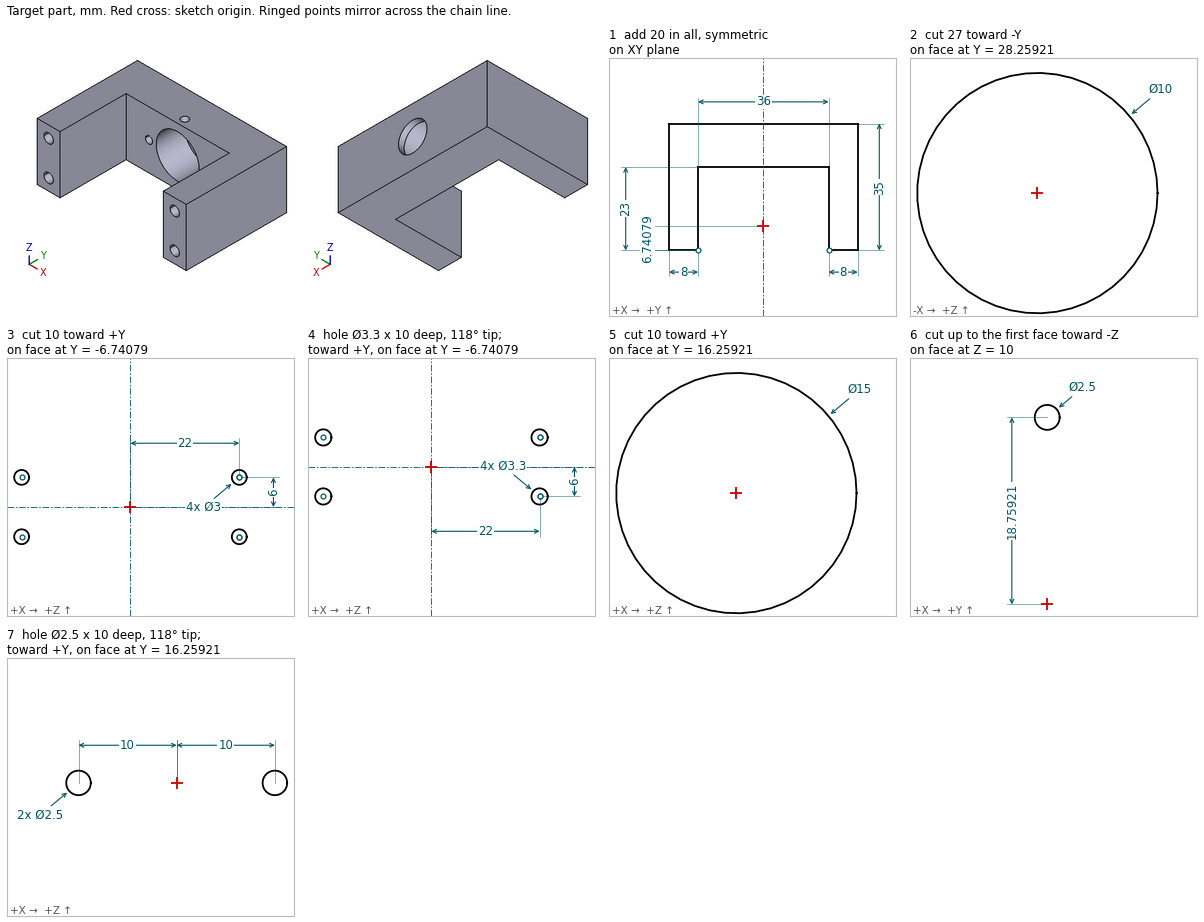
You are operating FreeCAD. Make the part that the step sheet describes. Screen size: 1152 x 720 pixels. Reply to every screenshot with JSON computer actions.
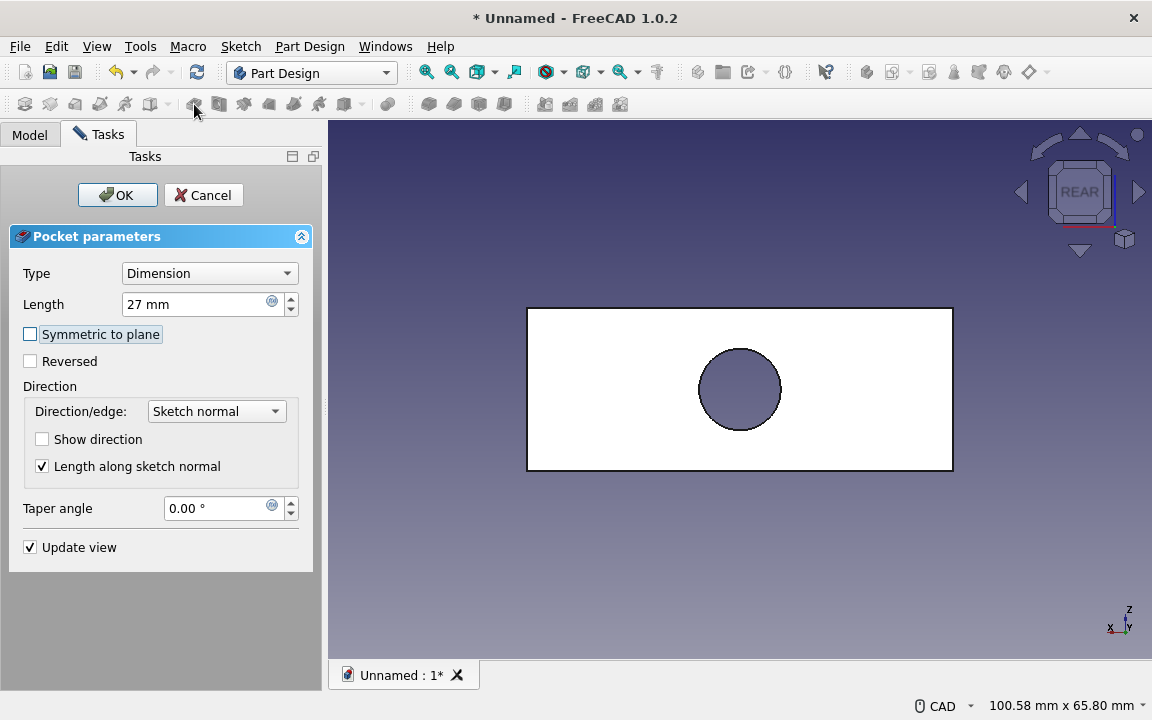
{"action": "left_click", "coordinate": [118, 195]}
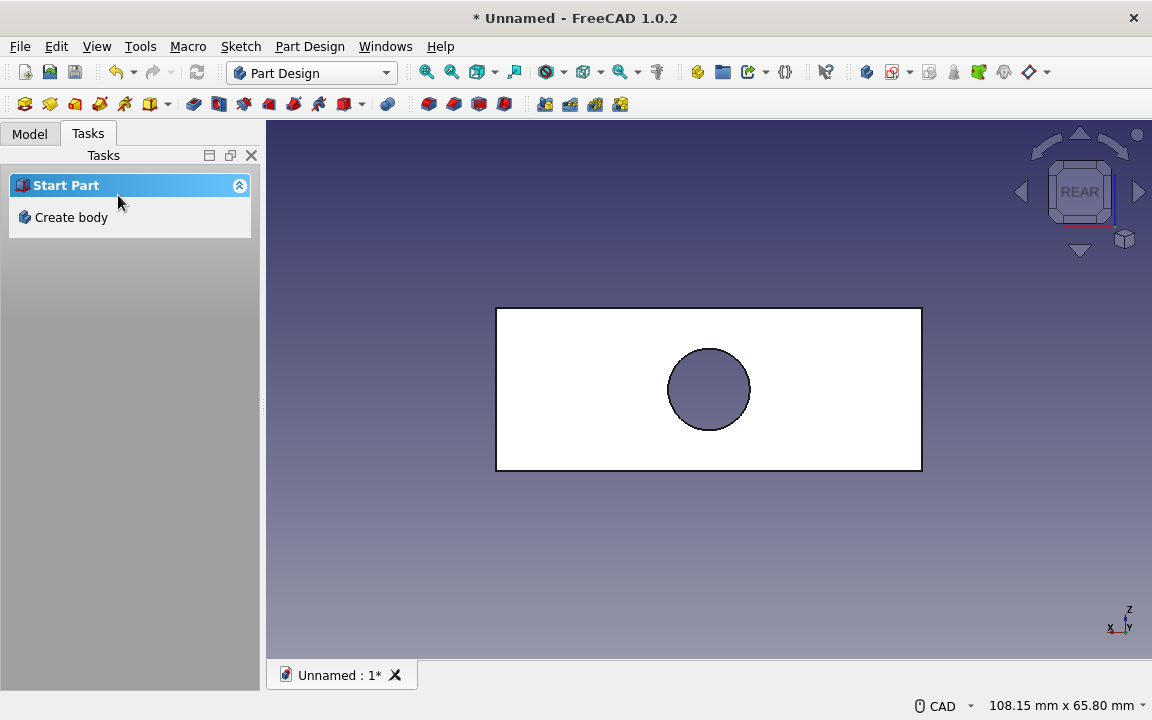
{"action": "key", "text": "0"}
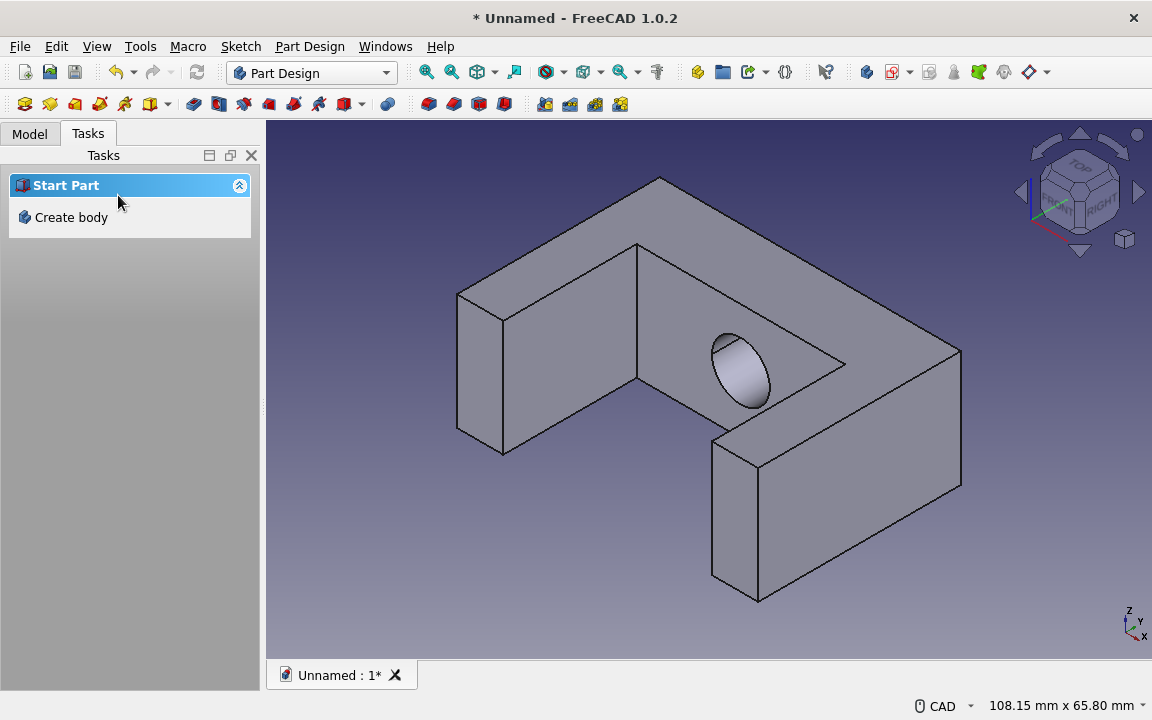
{"action": "left_click", "coordinate": [735, 482]}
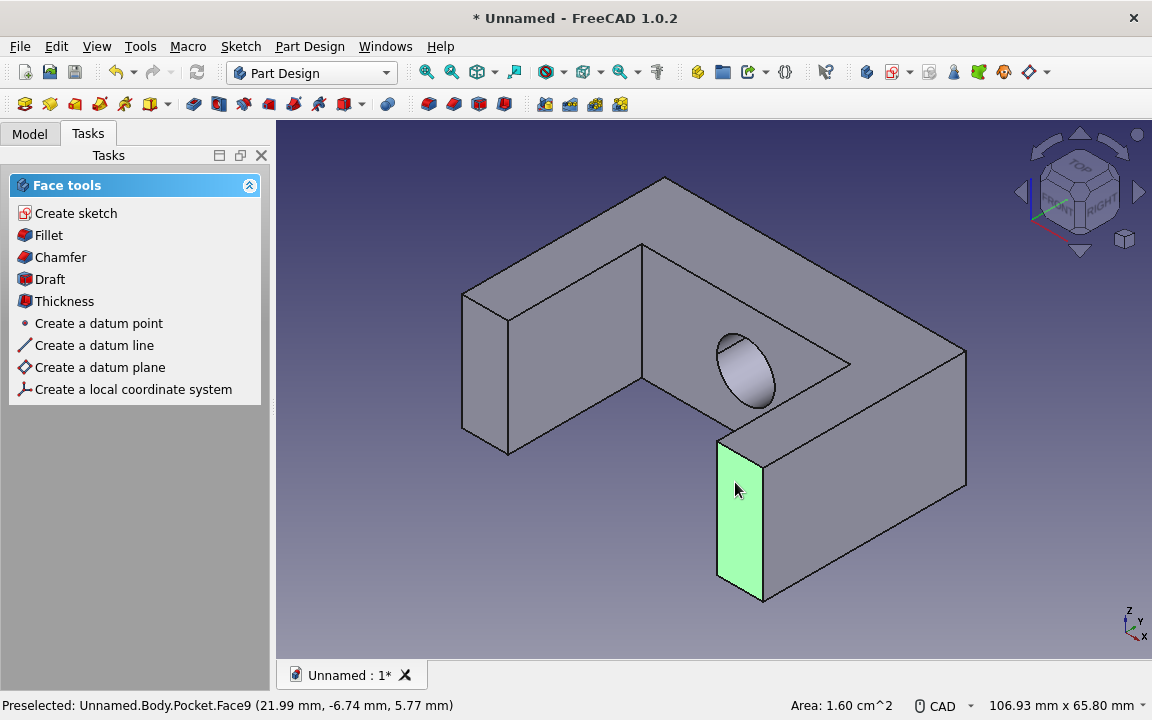
{"action": "left_click", "coordinate": [892, 72]}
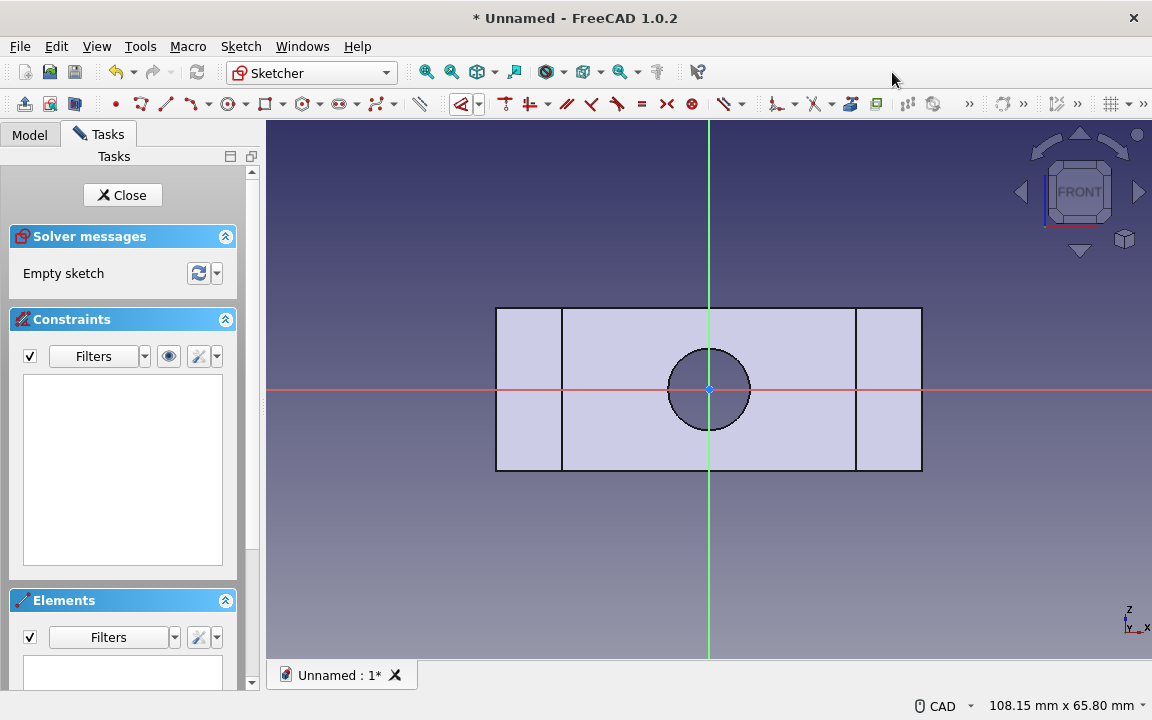
{"action": "key", "text": "g c"}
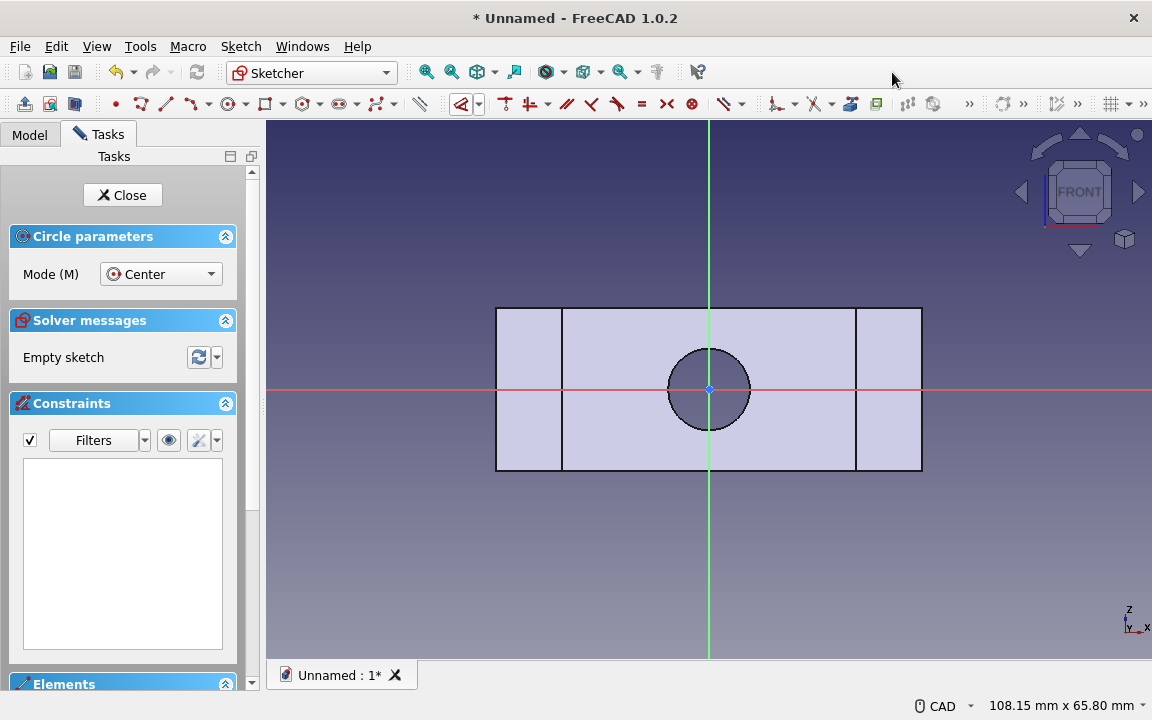
{"action": "scroll", "coordinate": [889, 340], "scroll_direction": "up", "scroll_amount": 4}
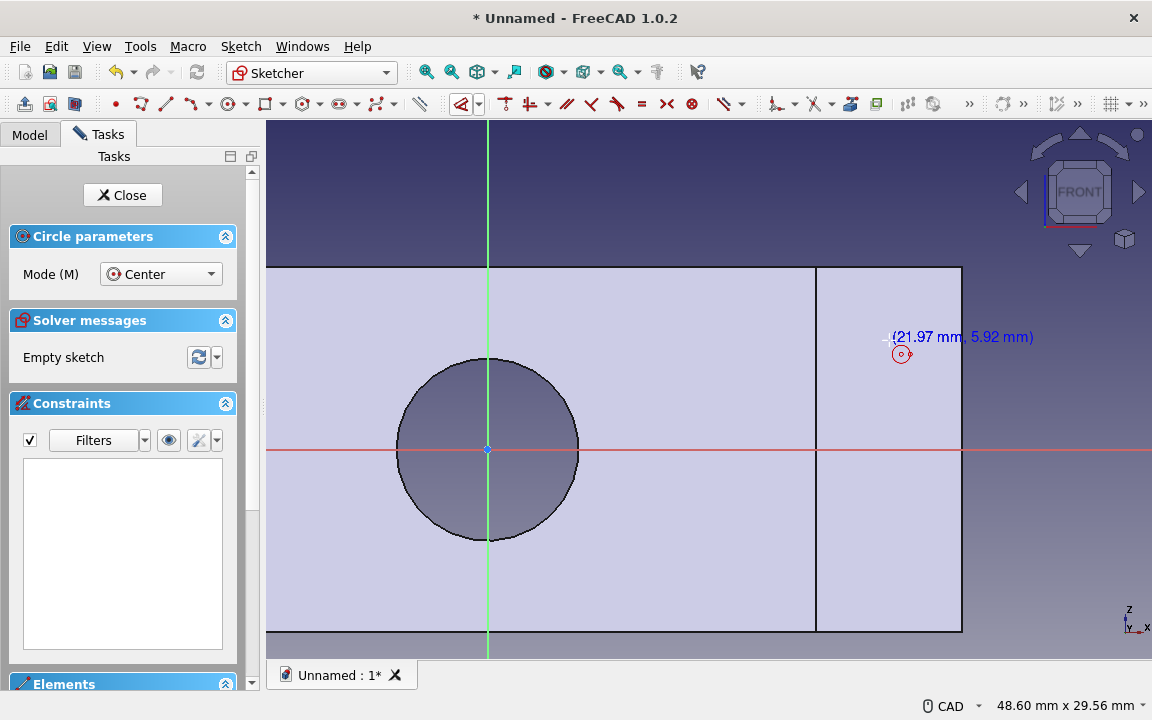
{"action": "left_click", "coordinate": [889, 340]}
{"action": "left_click", "coordinate": [908, 321]}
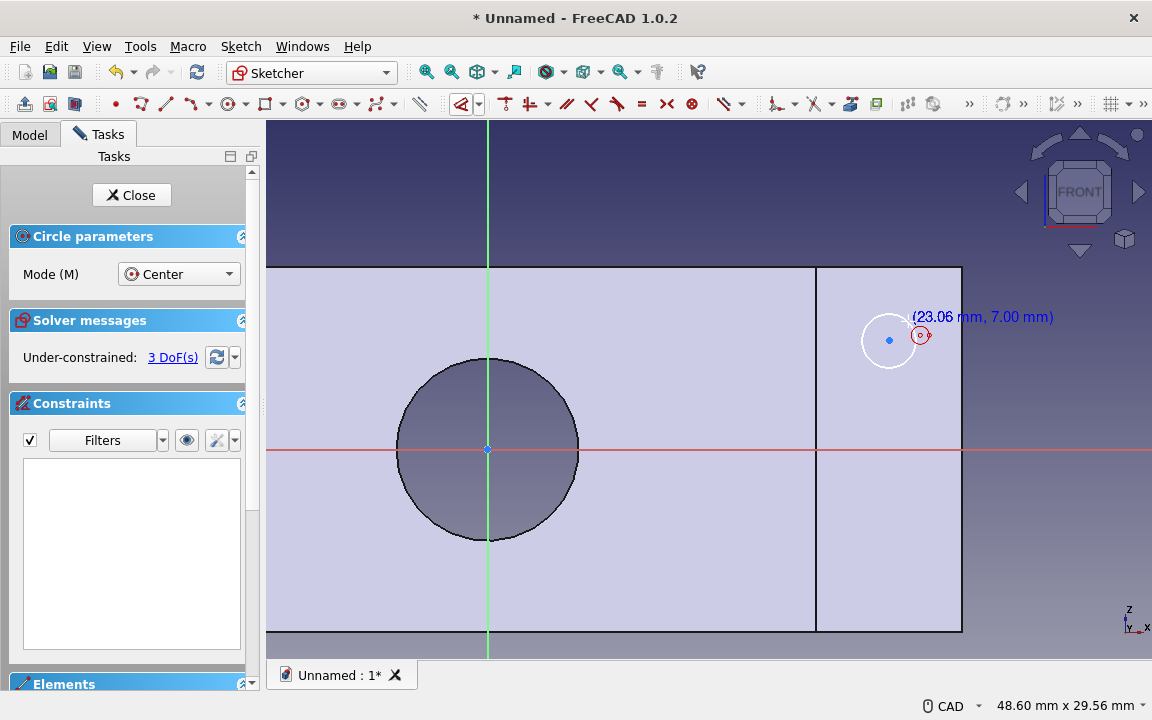
{"action": "left_click", "coordinate": [889, 559]}
{"action": "left_click", "coordinate": [908, 540]}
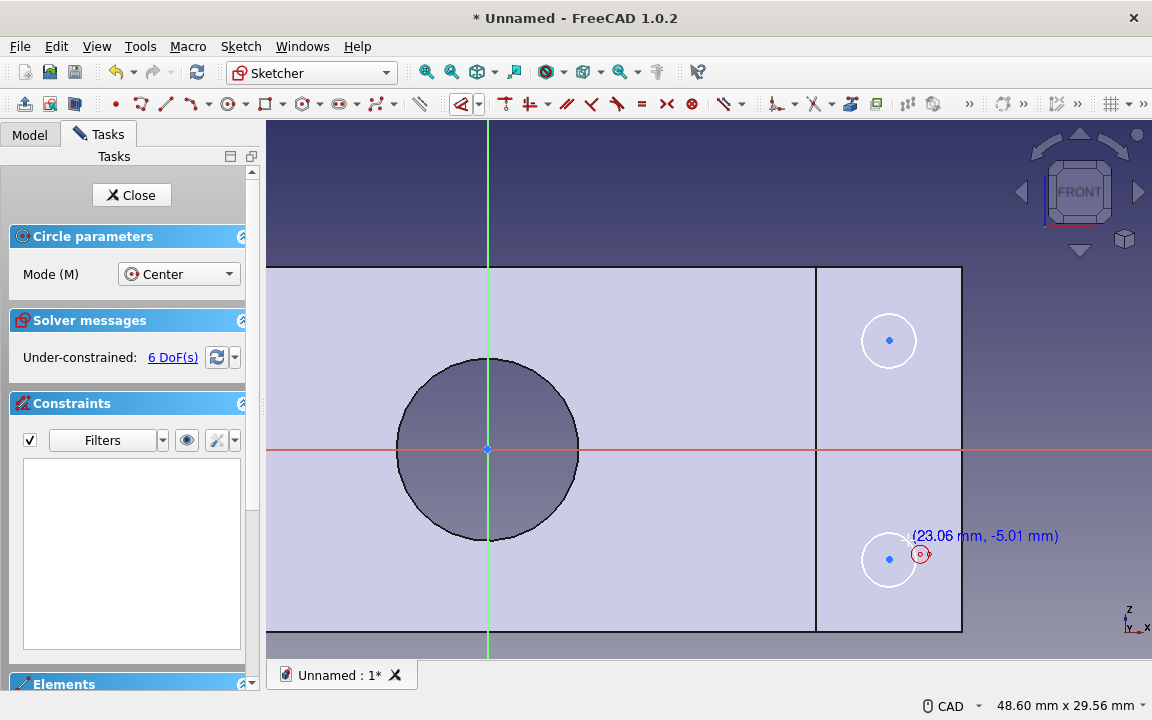
{"action": "scroll", "coordinate": [827, 316], "scroll_direction": "down", "scroll_amount": 3}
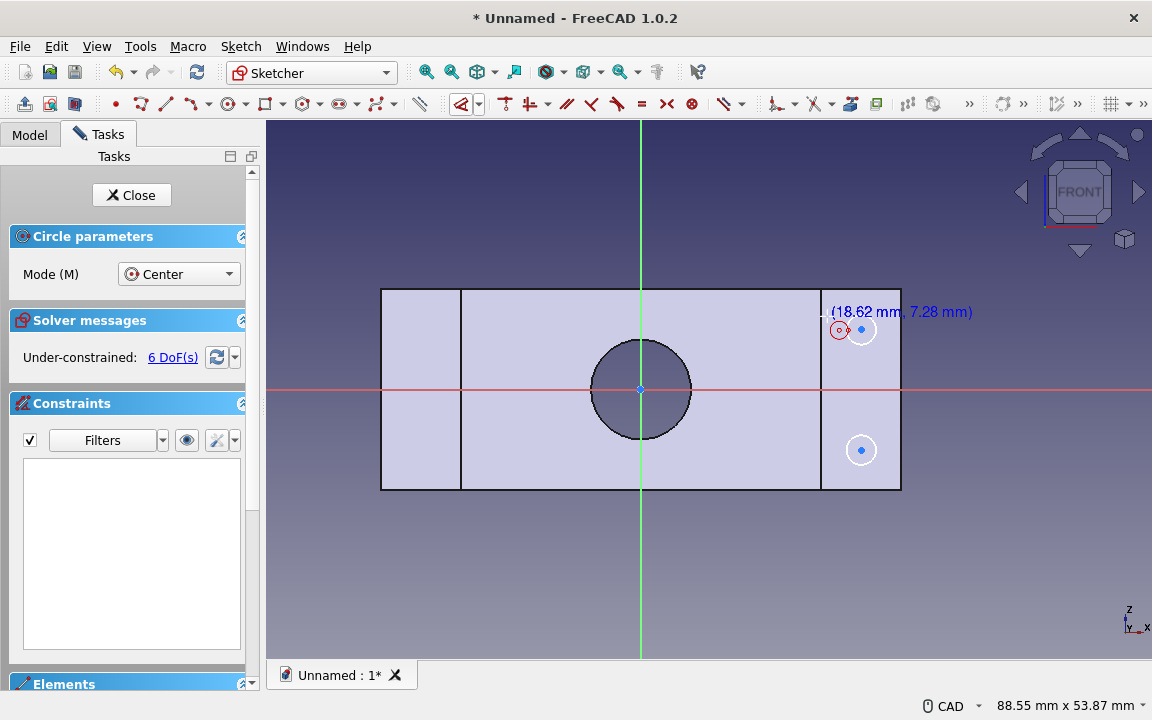
{"action": "scroll", "coordinate": [421, 450], "scroll_direction": "up", "scroll_amount": 3}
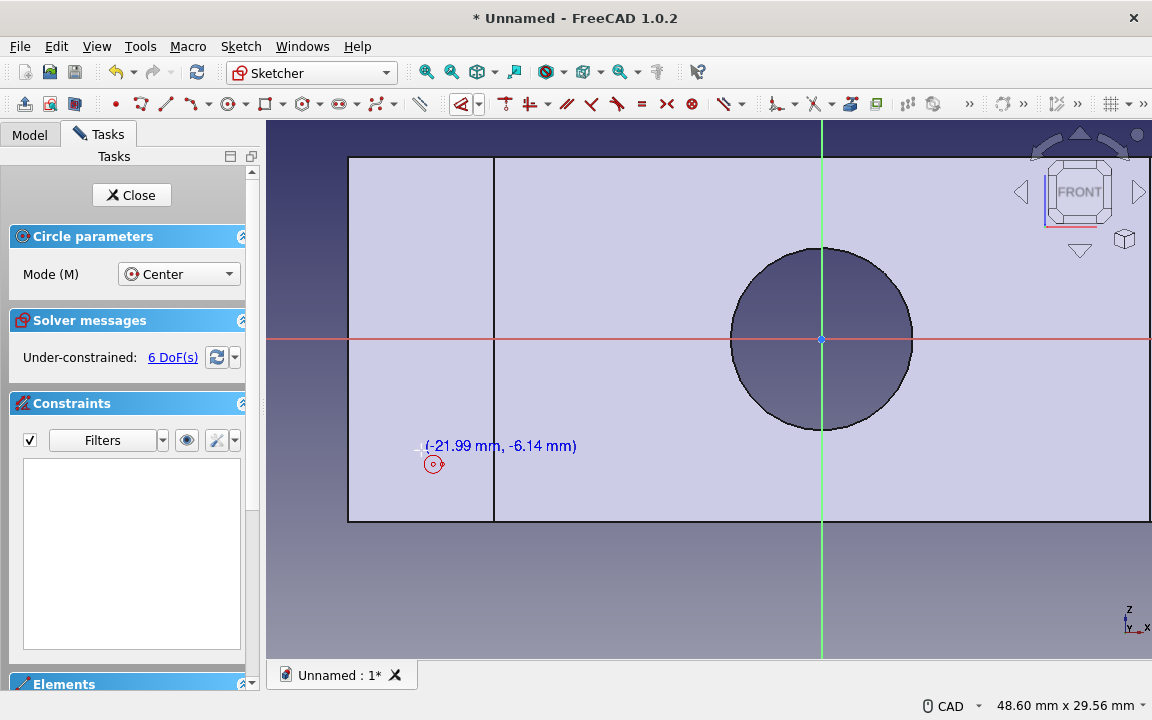
{"action": "left_click", "coordinate": [421, 449]}
{"action": "left_click", "coordinate": [440, 429]}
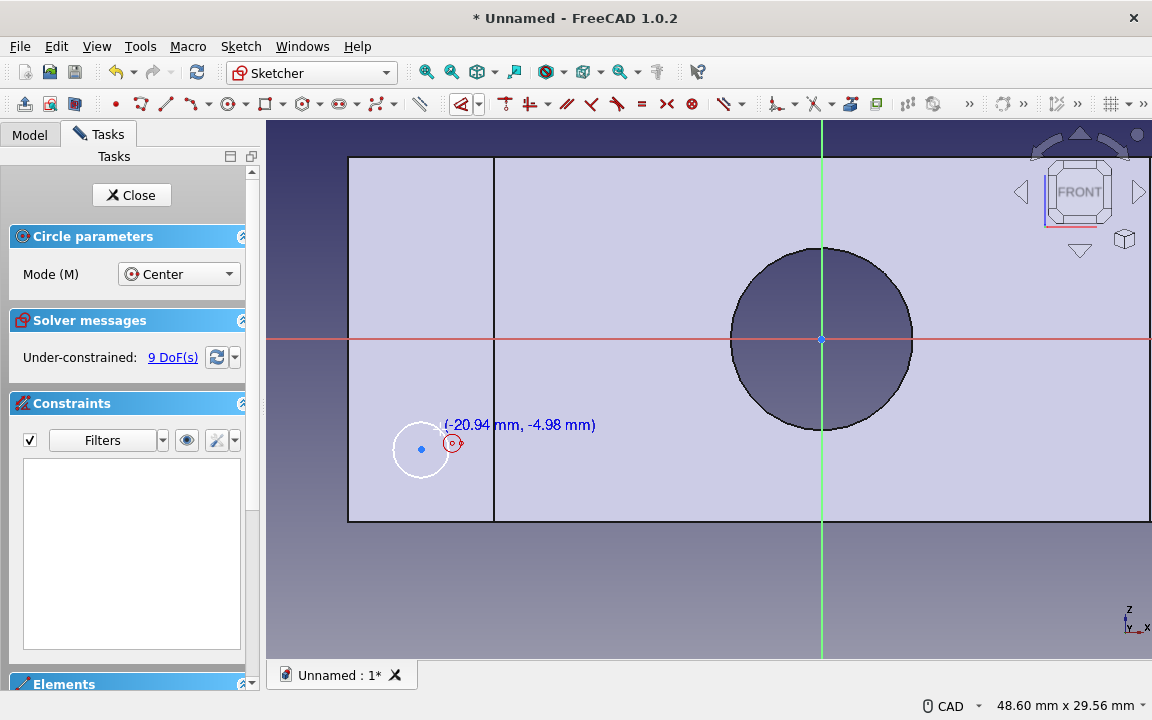
{"action": "left_click", "coordinate": [421, 230]}
{"action": "left_click", "coordinate": [440, 211]}
{"action": "key", "text": "Escape"}